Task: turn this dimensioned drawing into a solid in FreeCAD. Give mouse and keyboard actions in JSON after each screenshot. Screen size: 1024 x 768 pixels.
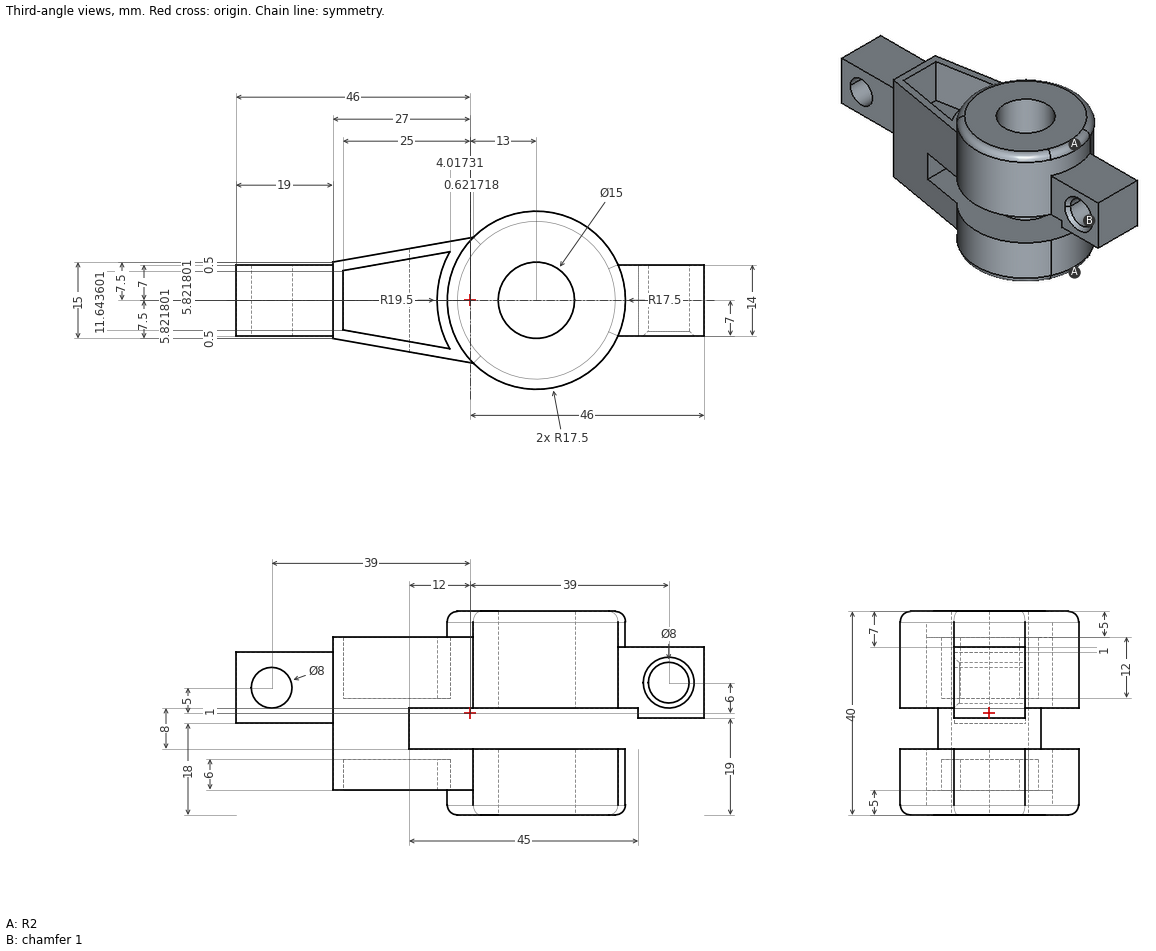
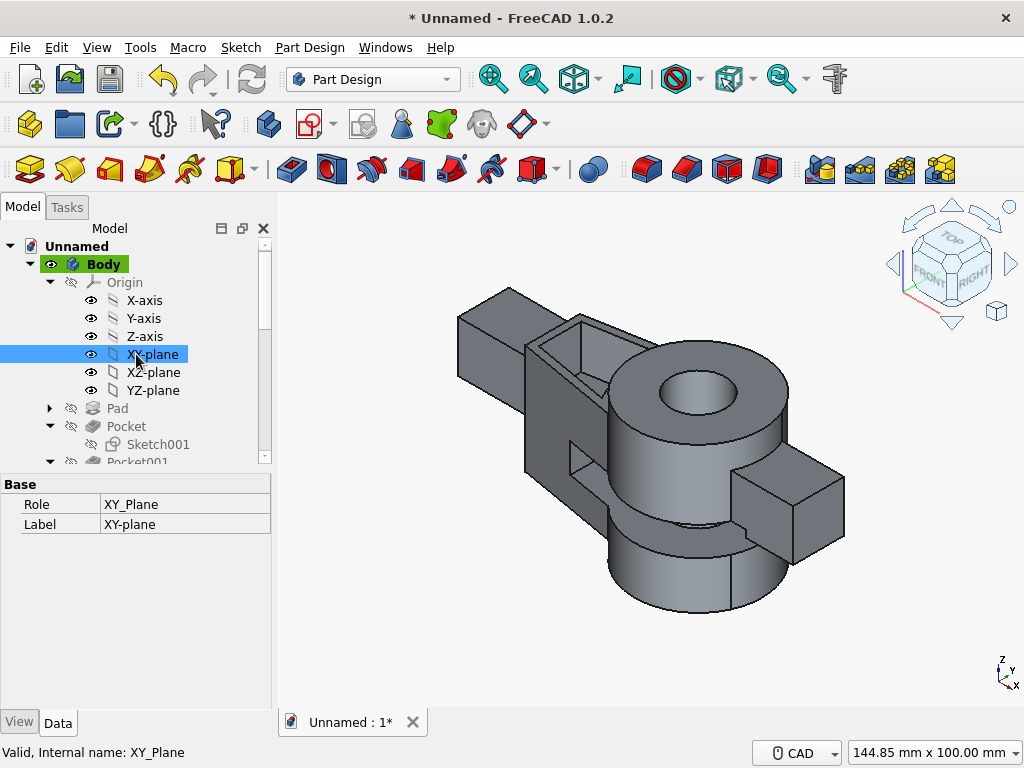
{"action": "left_click", "coordinate": [522, 124]}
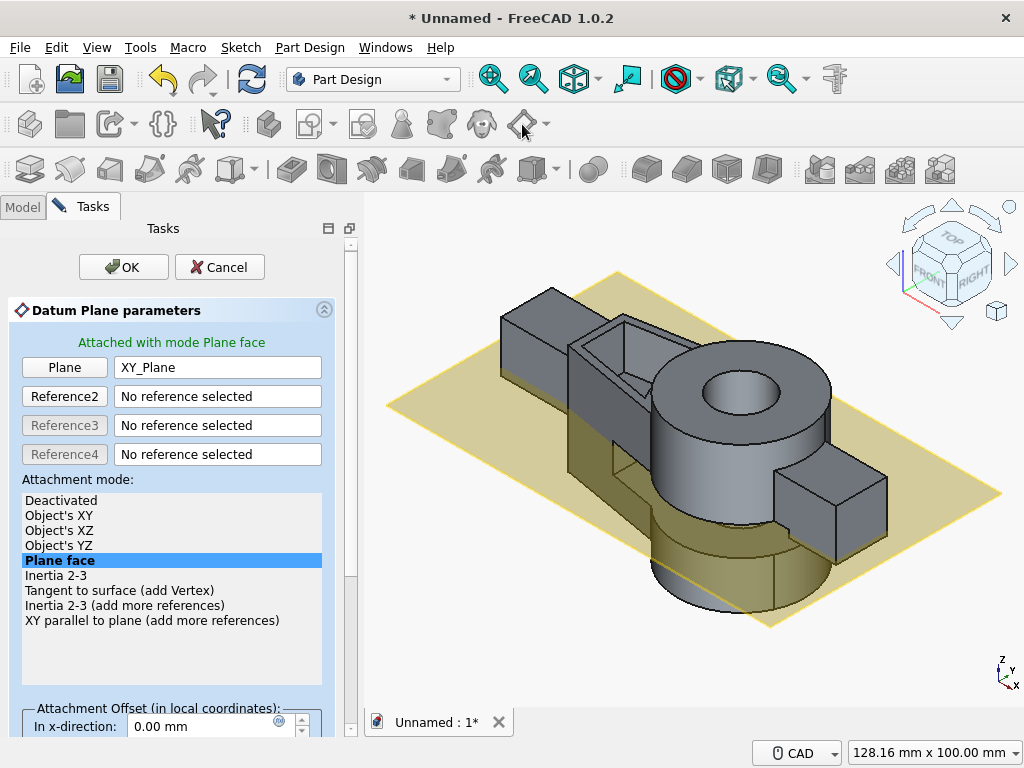
{"action": "scroll", "coordinate": [351, 487], "scroll_direction": "down", "scroll_amount": 3}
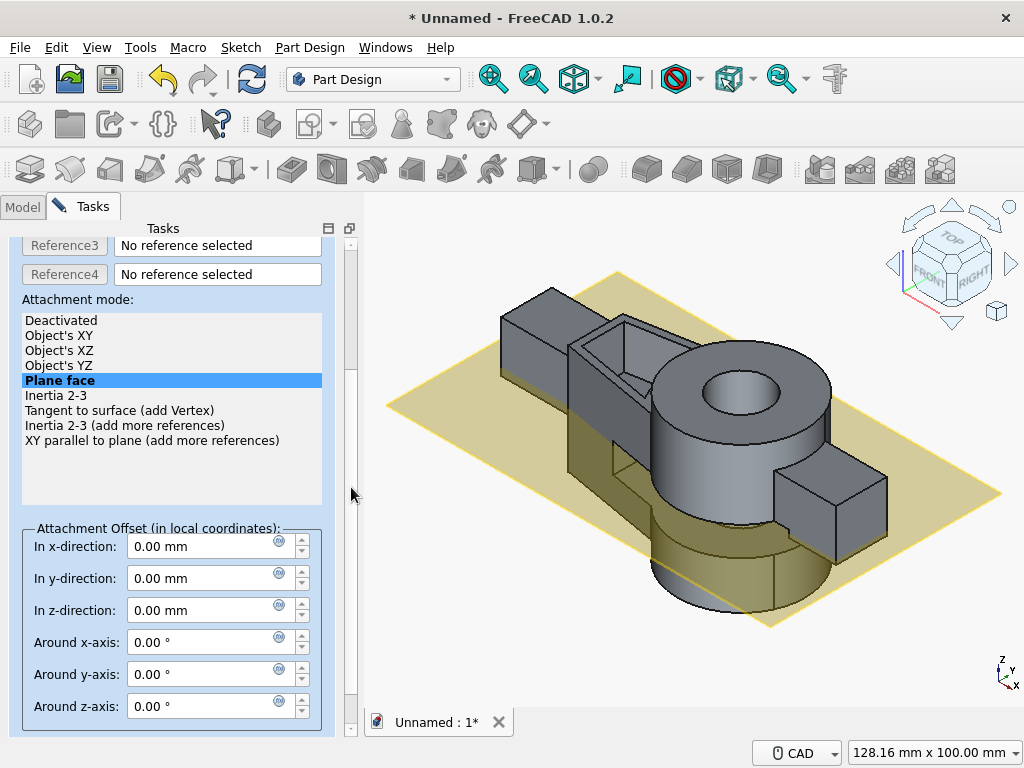
{"action": "triple_click", "coordinate": [210, 610]}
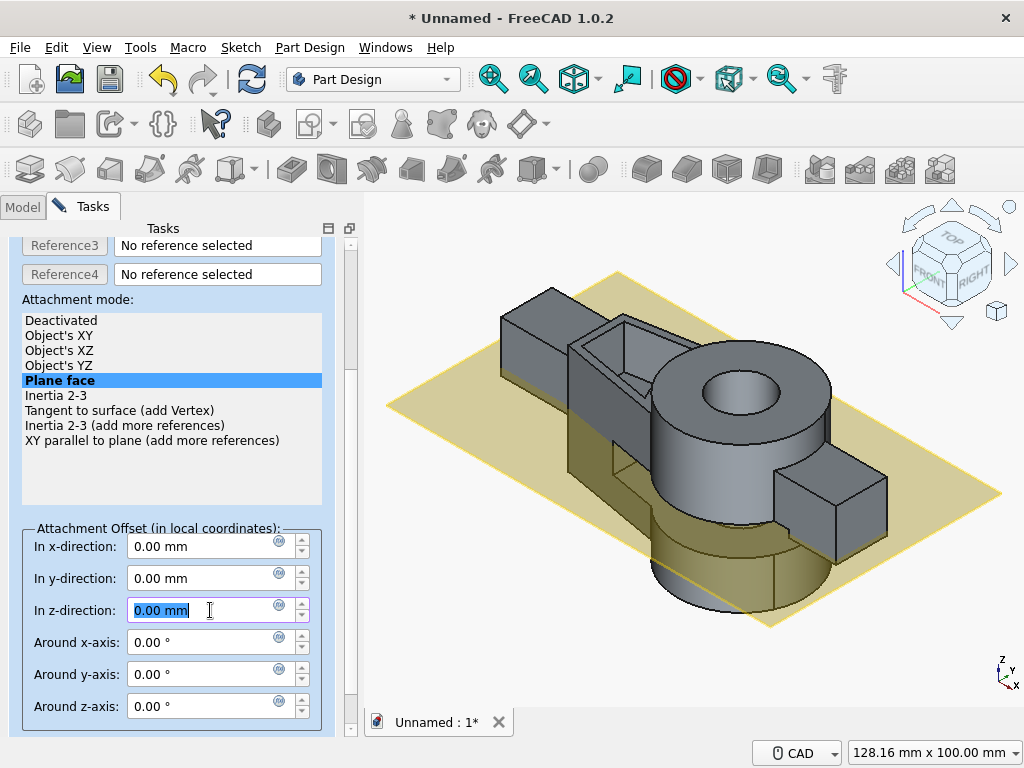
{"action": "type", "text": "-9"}
{"action": "key", "text": "Tab"}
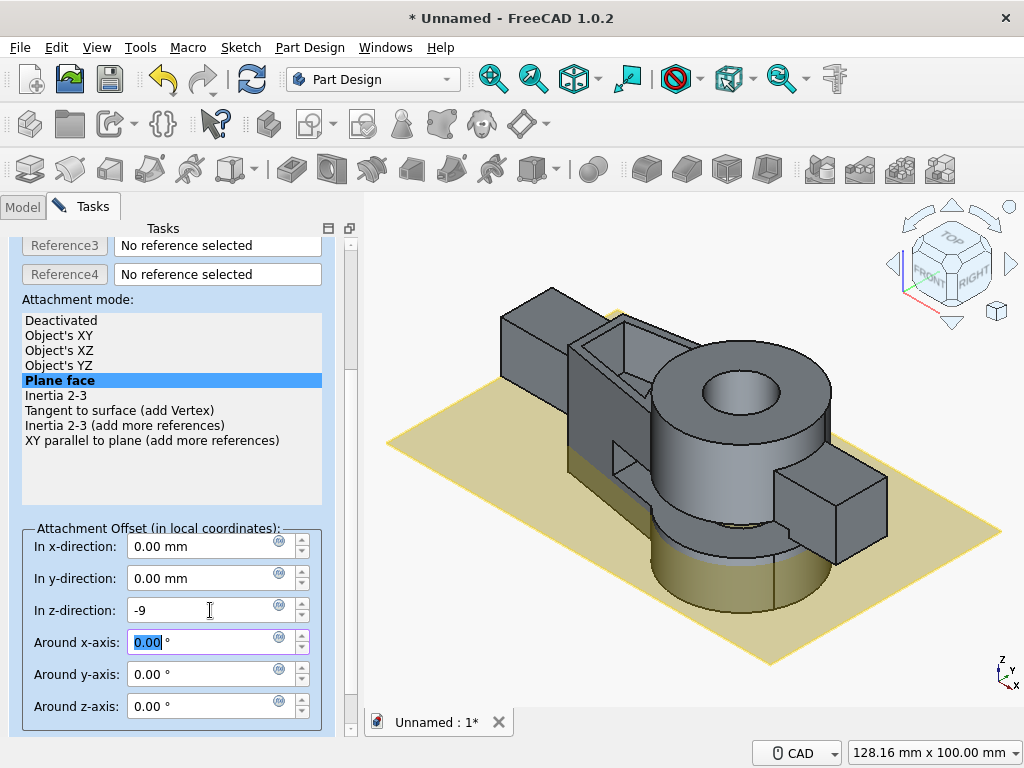
{"action": "scroll", "coordinate": [351, 487], "scroll_direction": "up", "scroll_amount": 4}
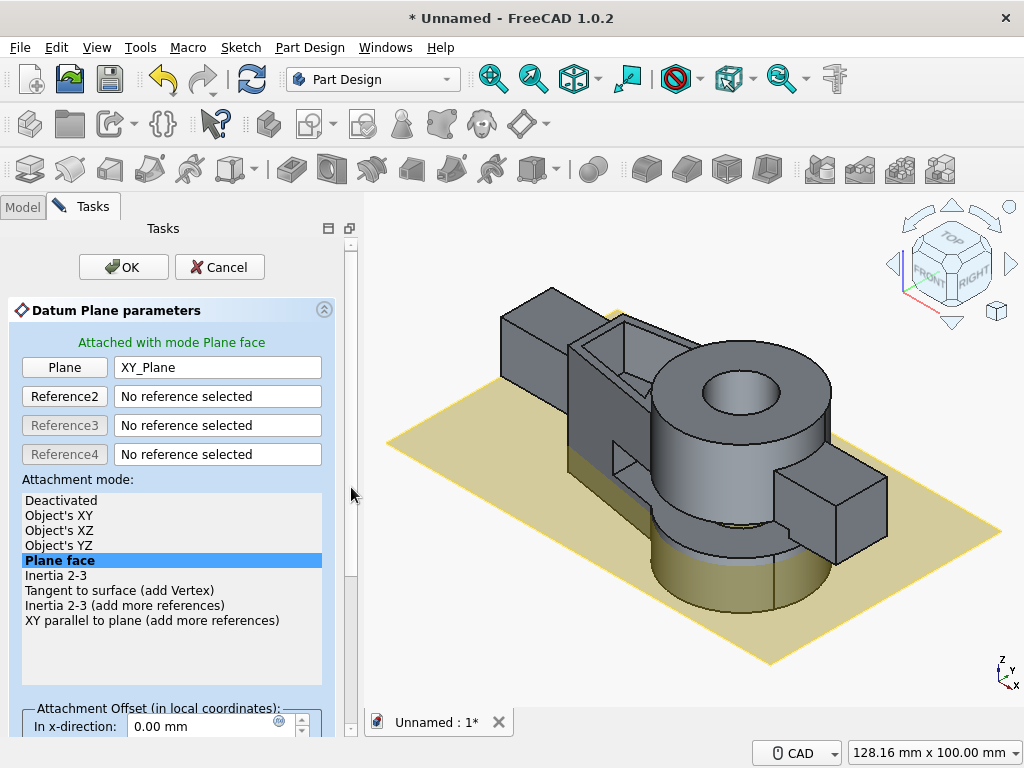
{"action": "left_click", "coordinate": [124, 267]}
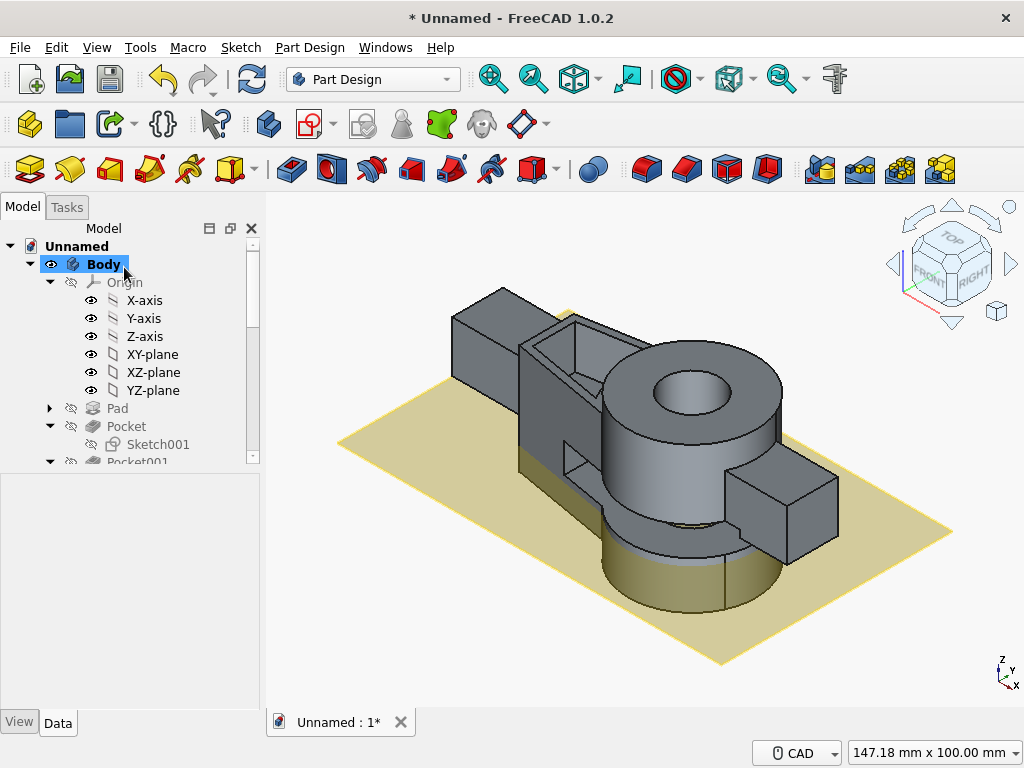
{"action": "scroll", "coordinate": [100, 350], "scroll_direction": "down", "scroll_amount": 3}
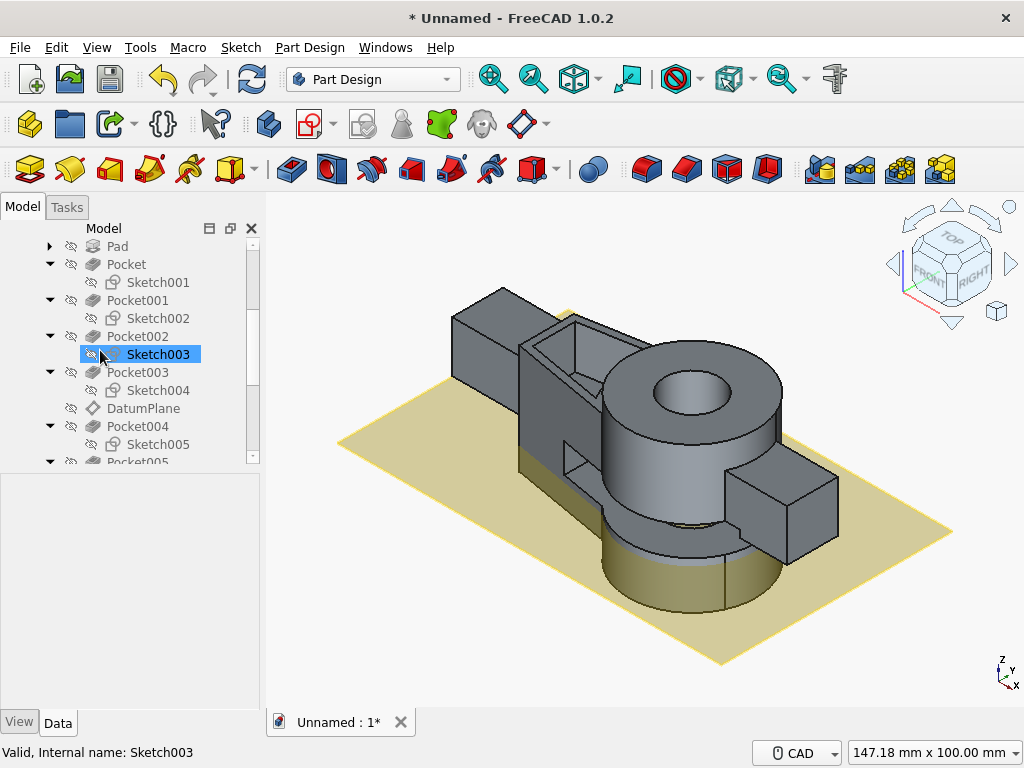
{"action": "scroll", "coordinate": [140, 350], "scroll_direction": "up", "scroll_amount": 15}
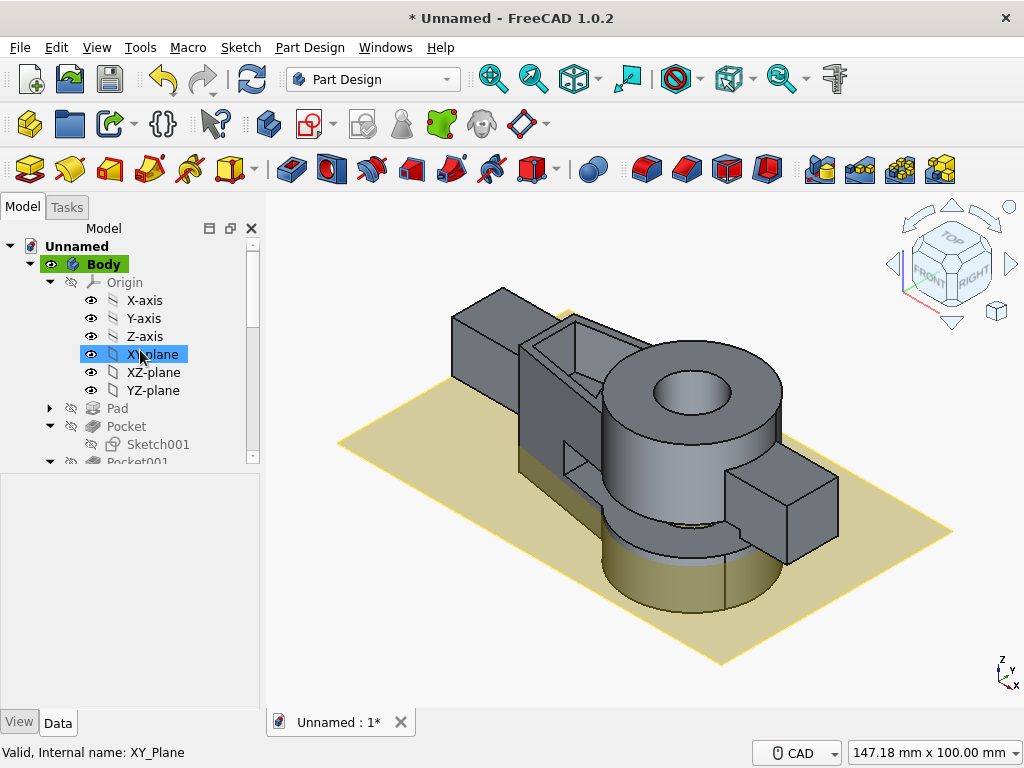
{"action": "scroll", "coordinate": [100, 350], "scroll_direction": "down", "scroll_amount": 6}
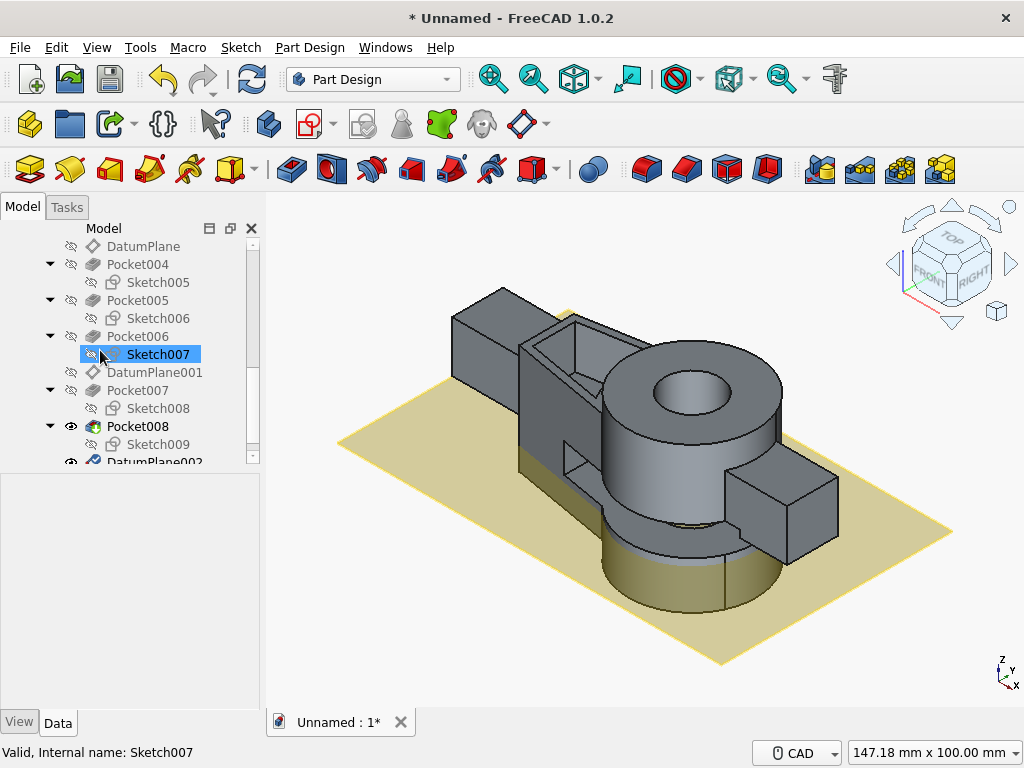
{"action": "left_click", "coordinate": [116, 462]}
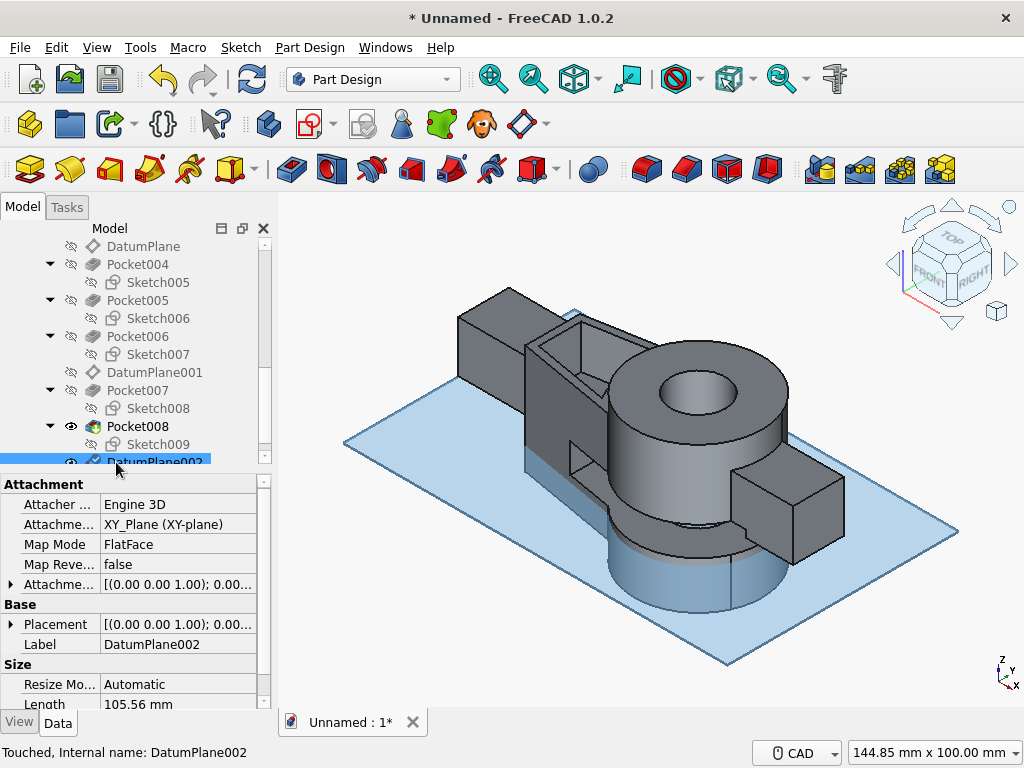
{"action": "left_click", "coordinate": [310, 124]}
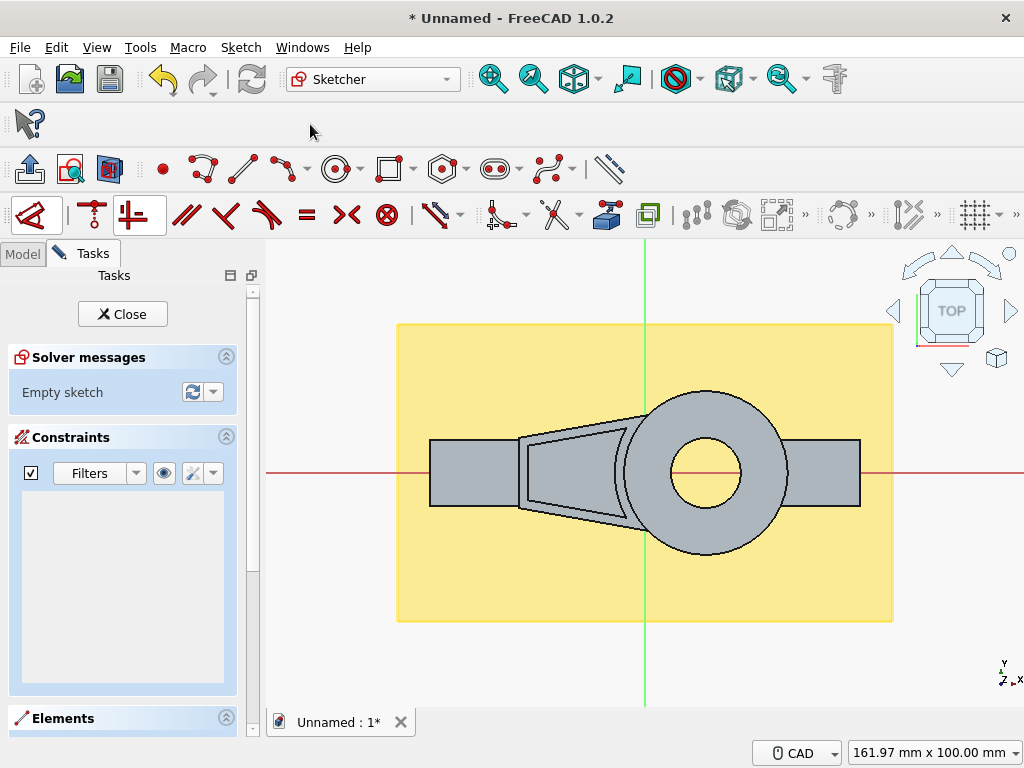
{"action": "left_click", "coordinate": [110, 170]}